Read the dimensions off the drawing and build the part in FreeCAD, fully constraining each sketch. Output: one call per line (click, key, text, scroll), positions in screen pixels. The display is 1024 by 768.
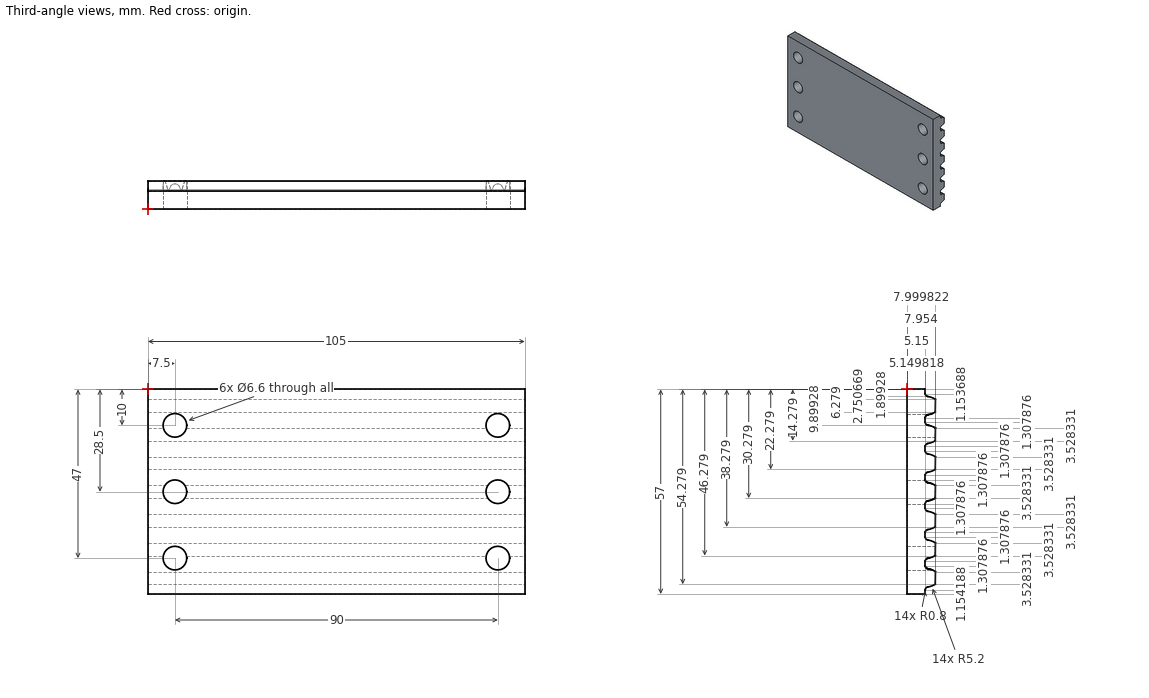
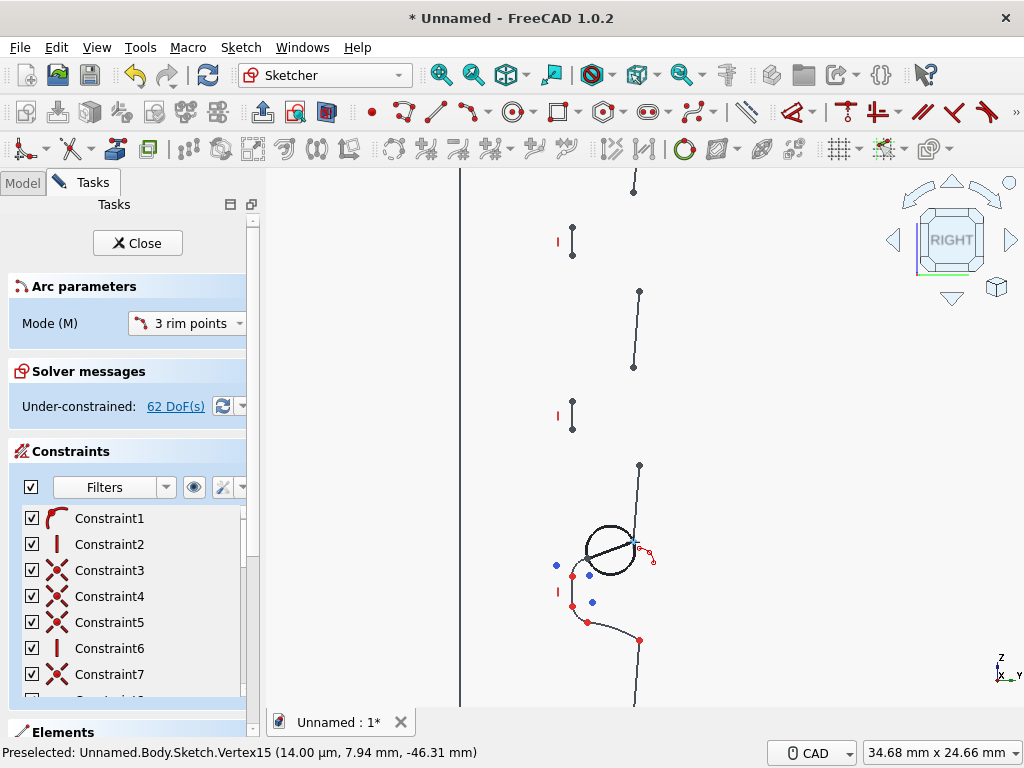
scroll(612, 552, up, 9)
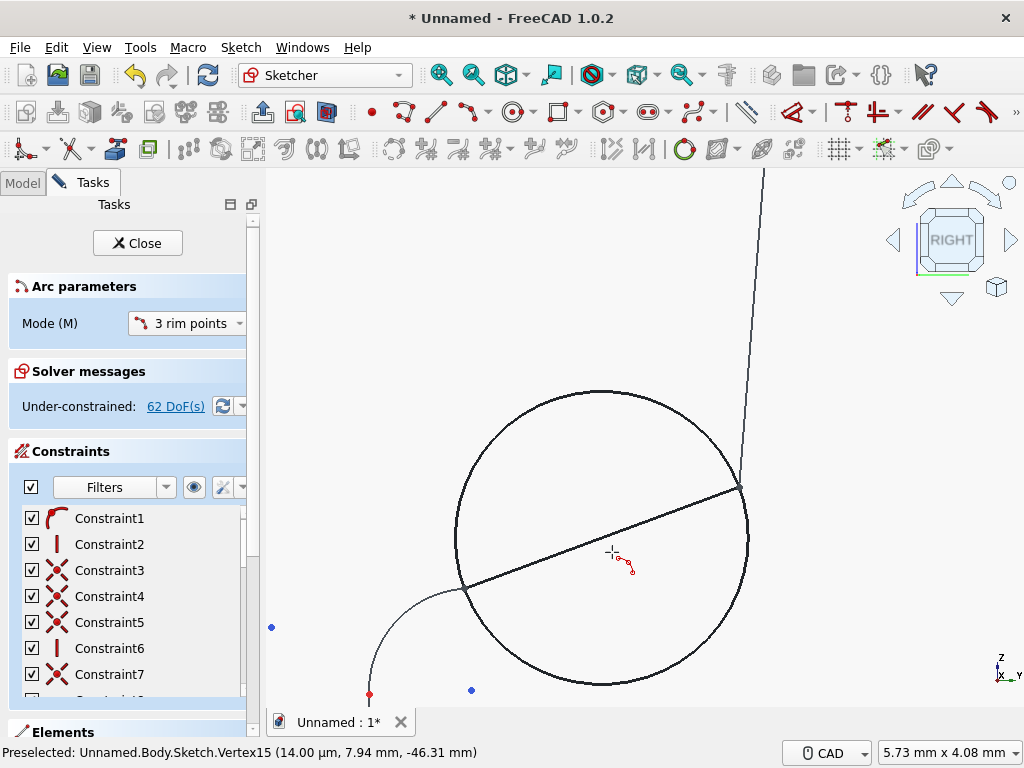
click(607, 549)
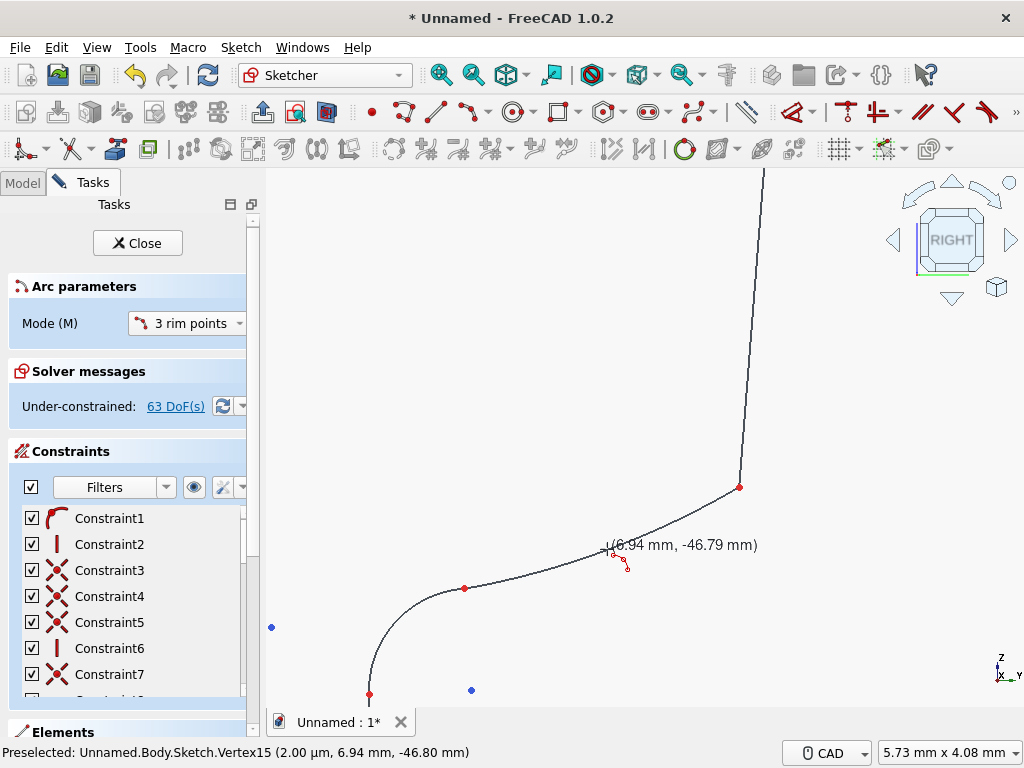
scroll(595, 558, down, 15)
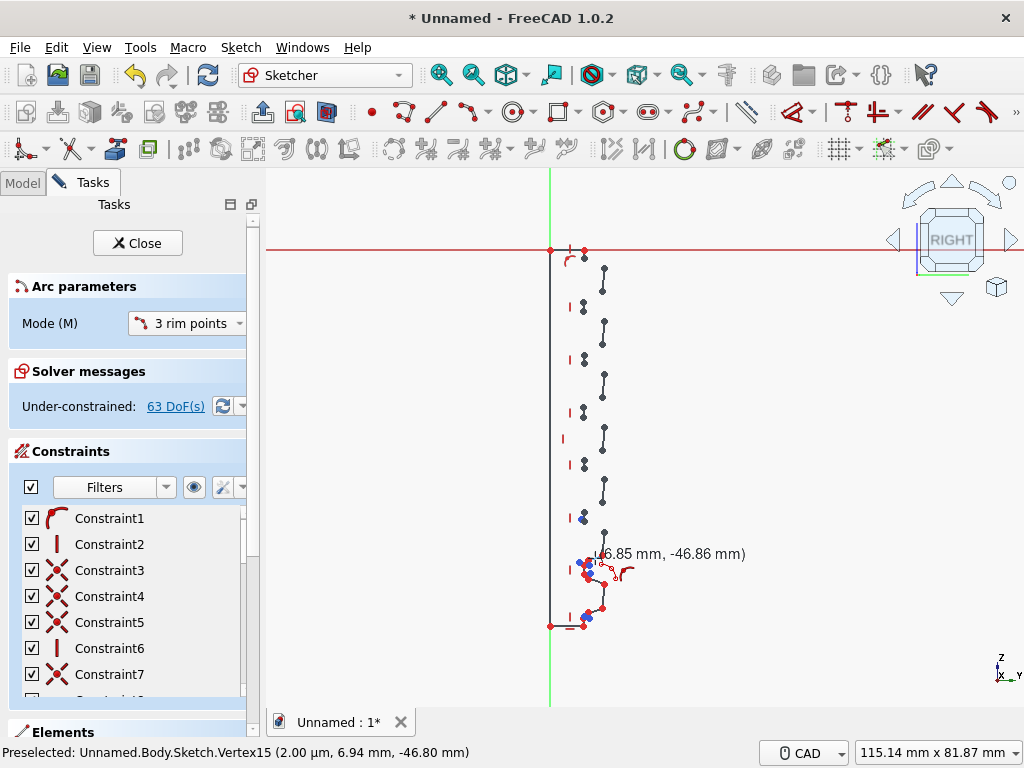
scroll(603, 532, up, 2)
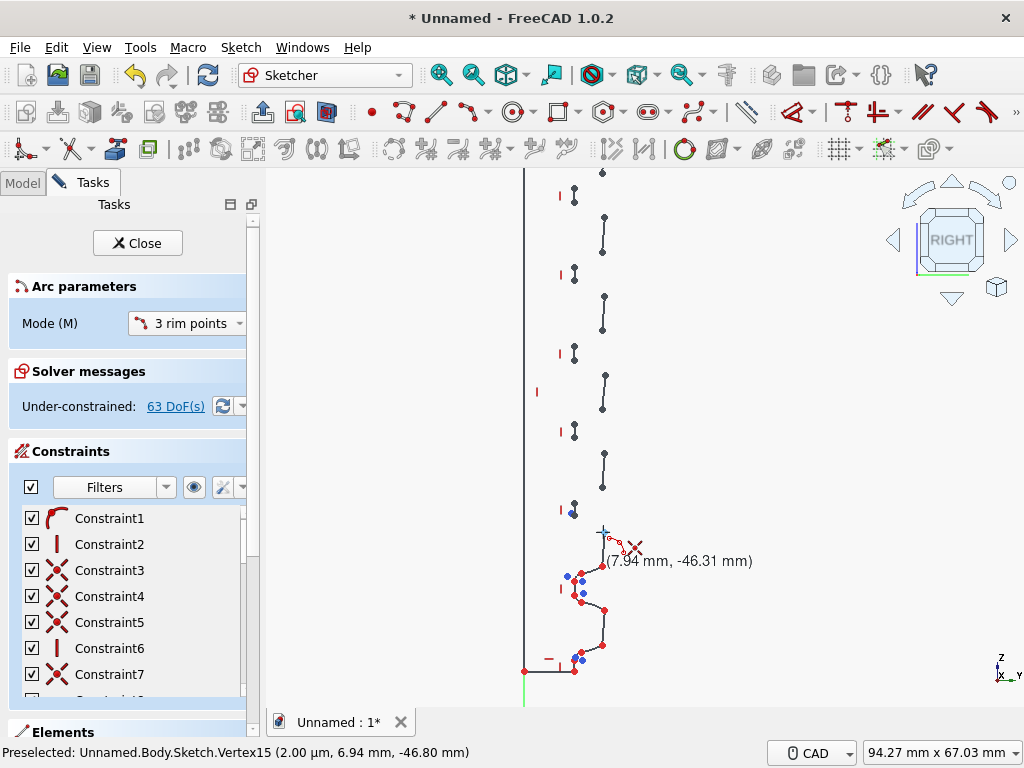
click(605, 532)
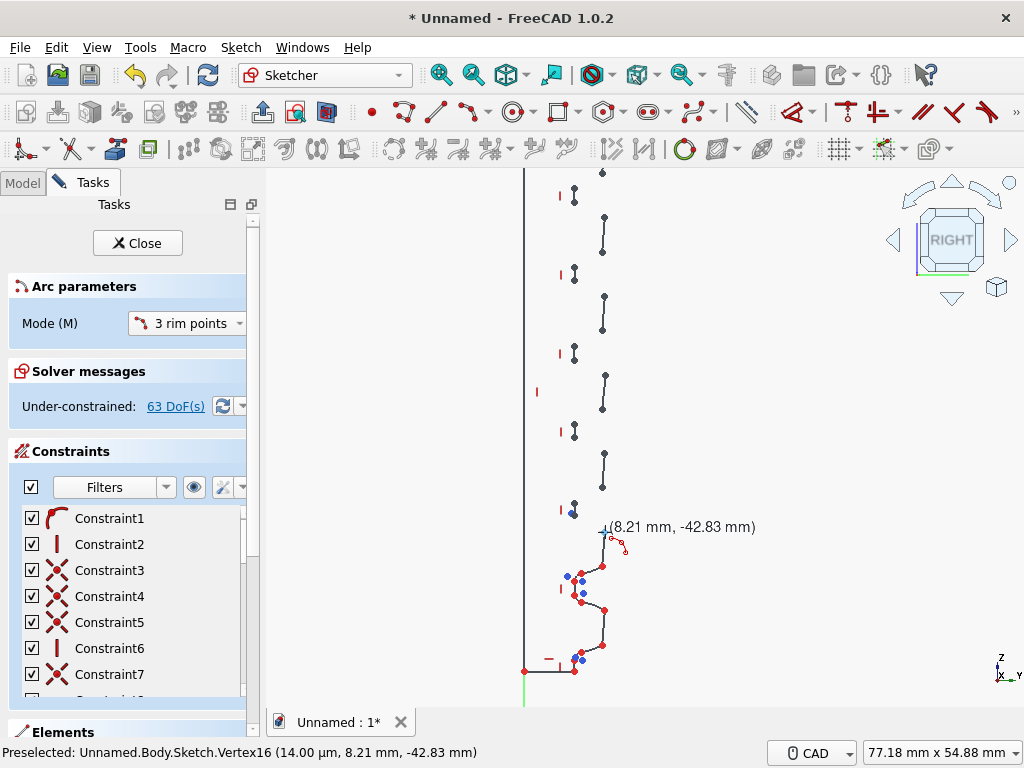
scroll(582, 523, up, 5)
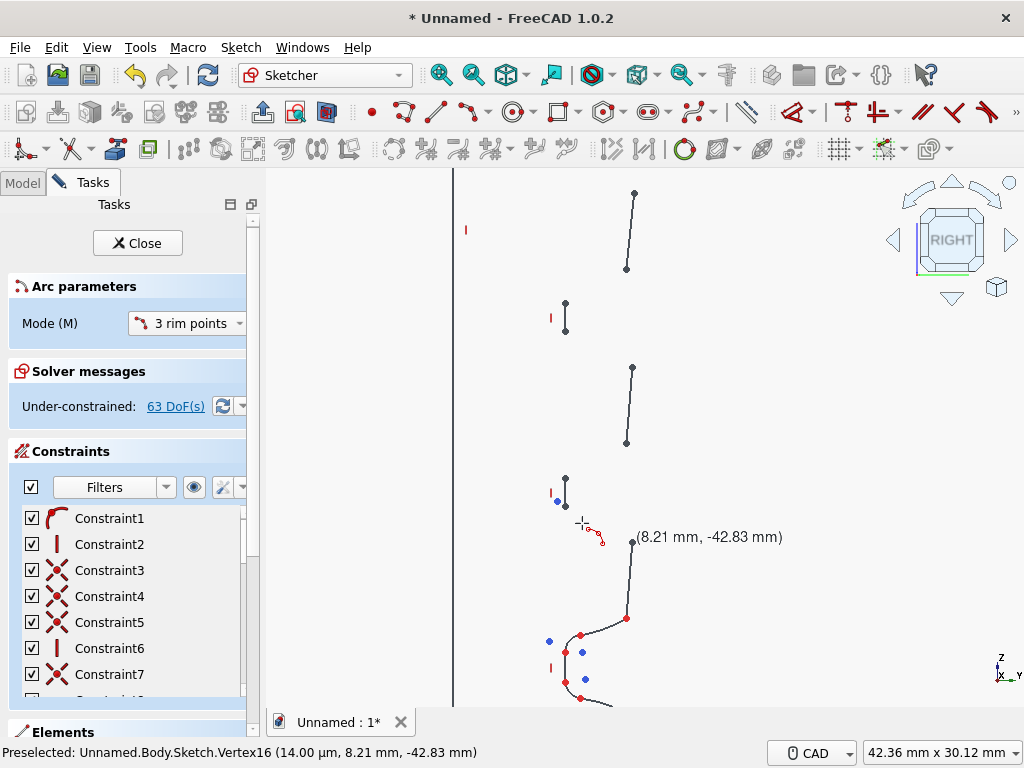
click(580, 523)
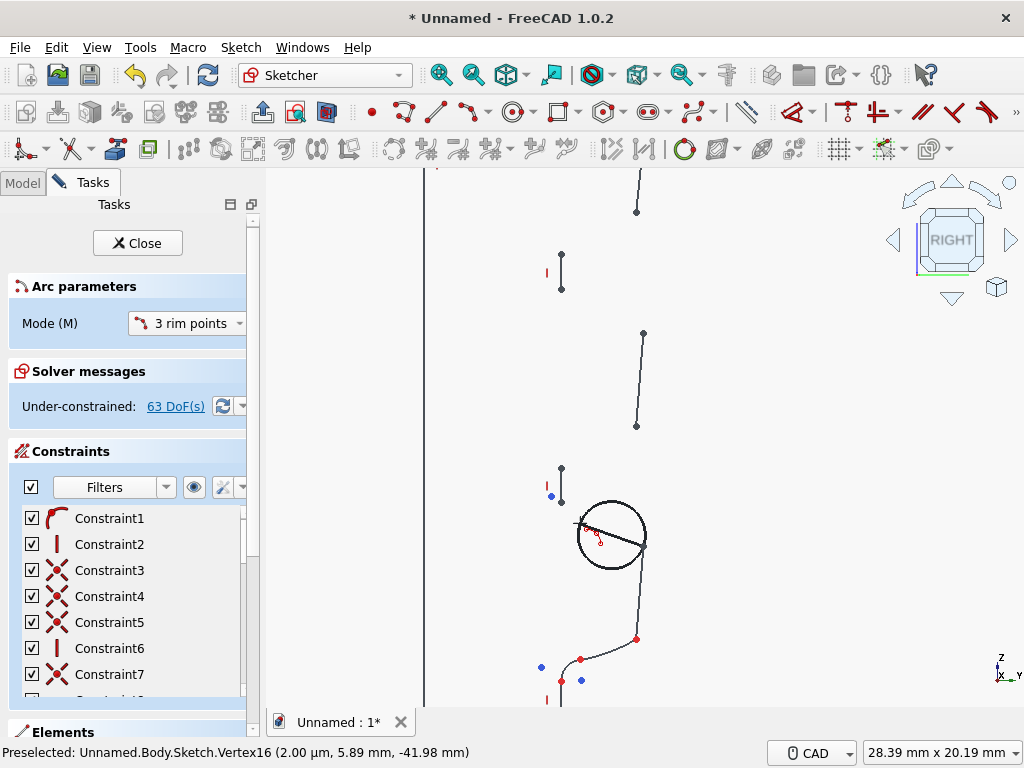
scroll(610, 530, up, 8)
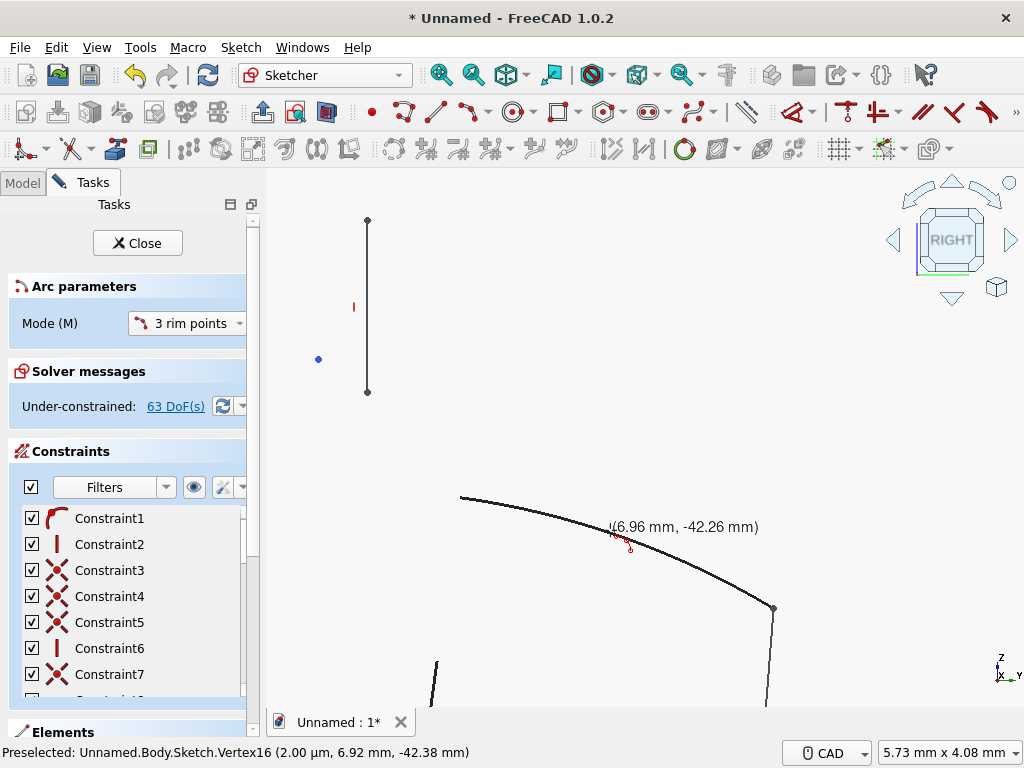
click(609, 529)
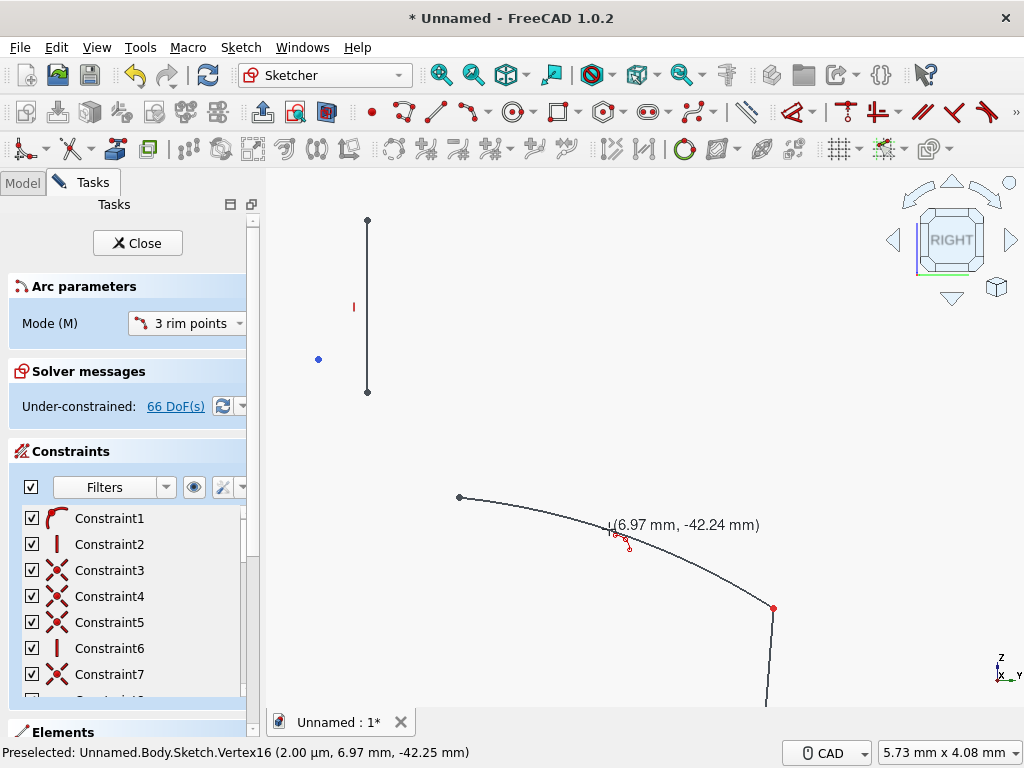
scroll(595, 528, down, 15)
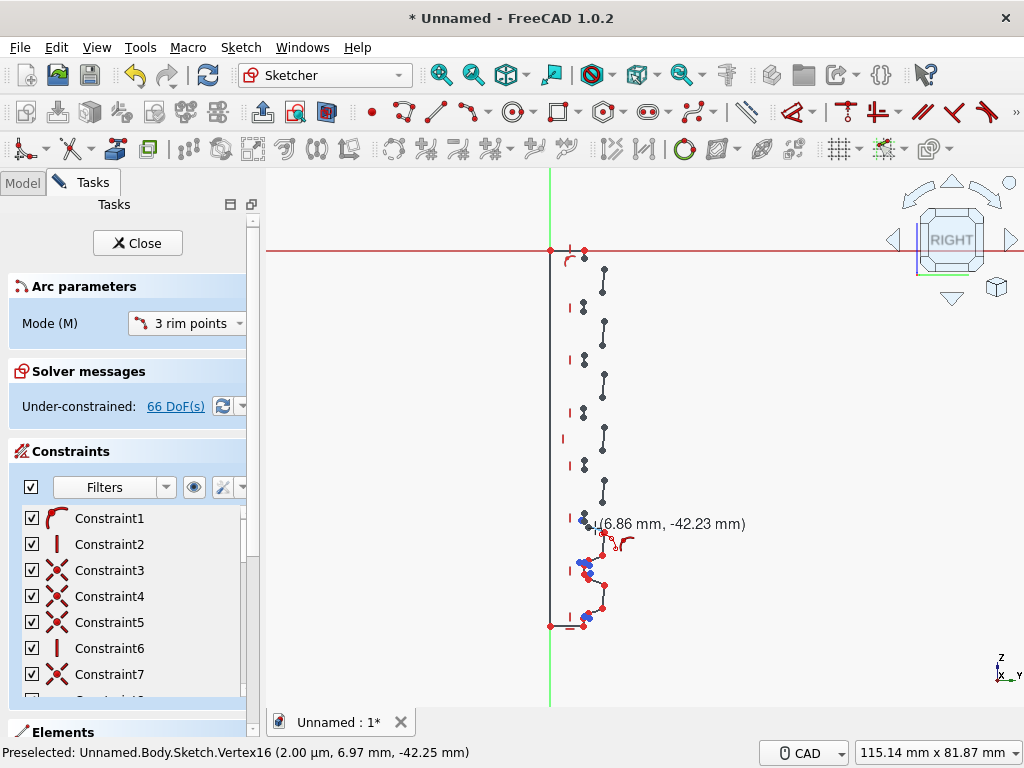
scroll(589, 527, up, 7)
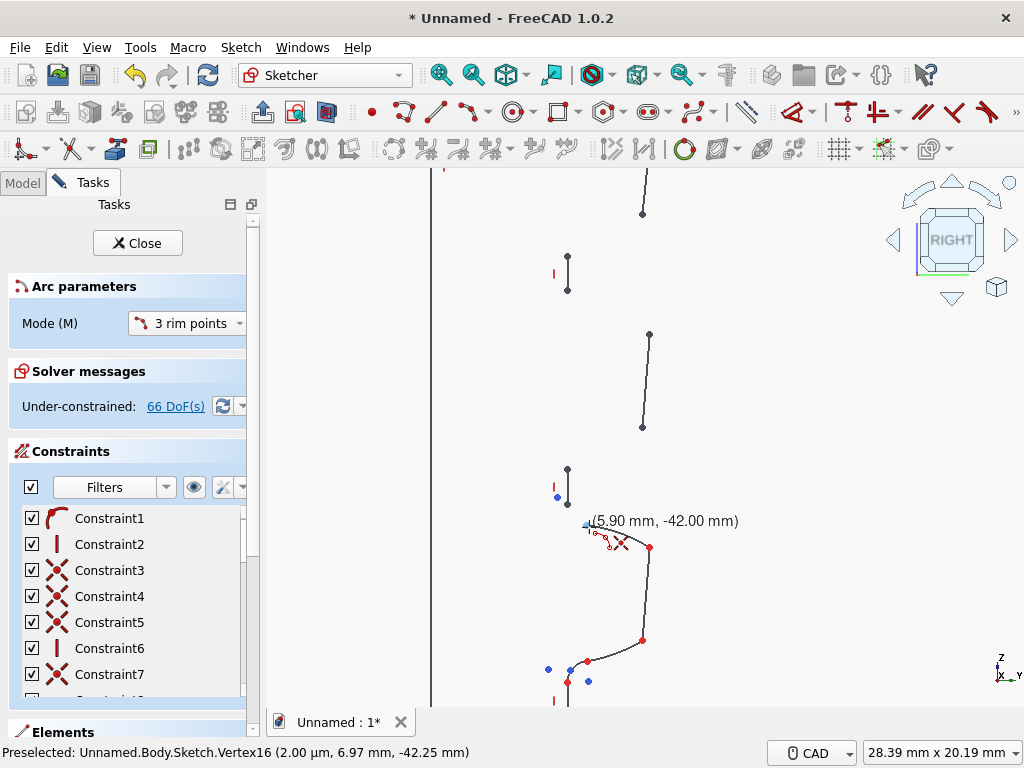
click(586, 525)
click(568, 504)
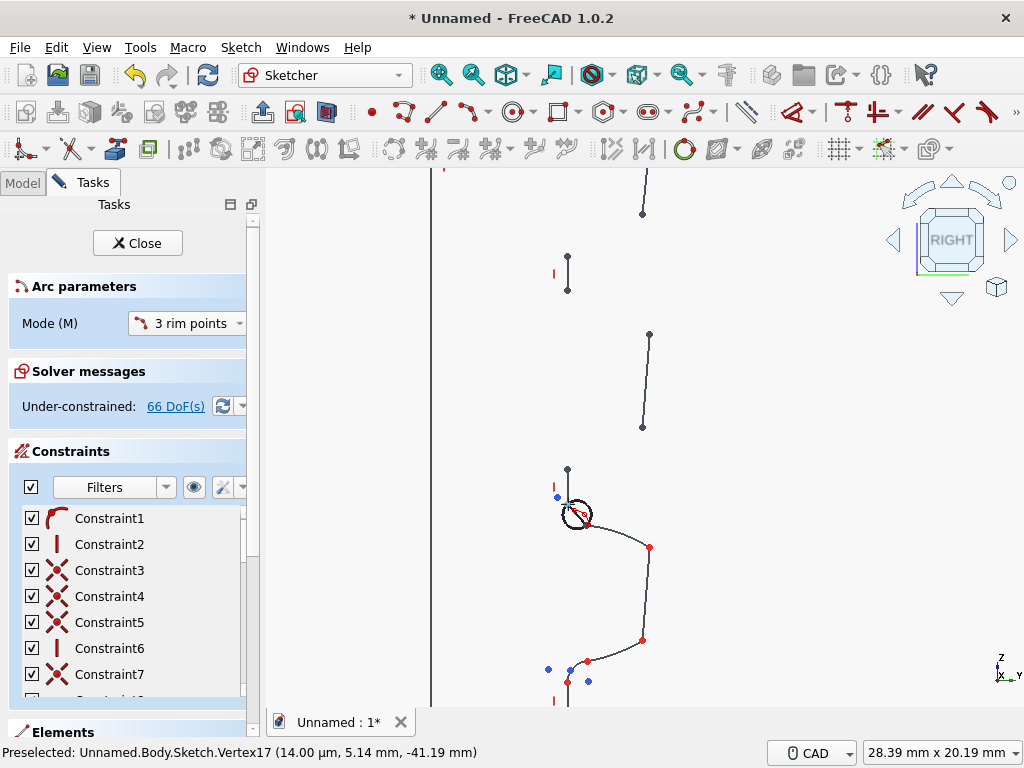
scroll(573, 517, up, 6)